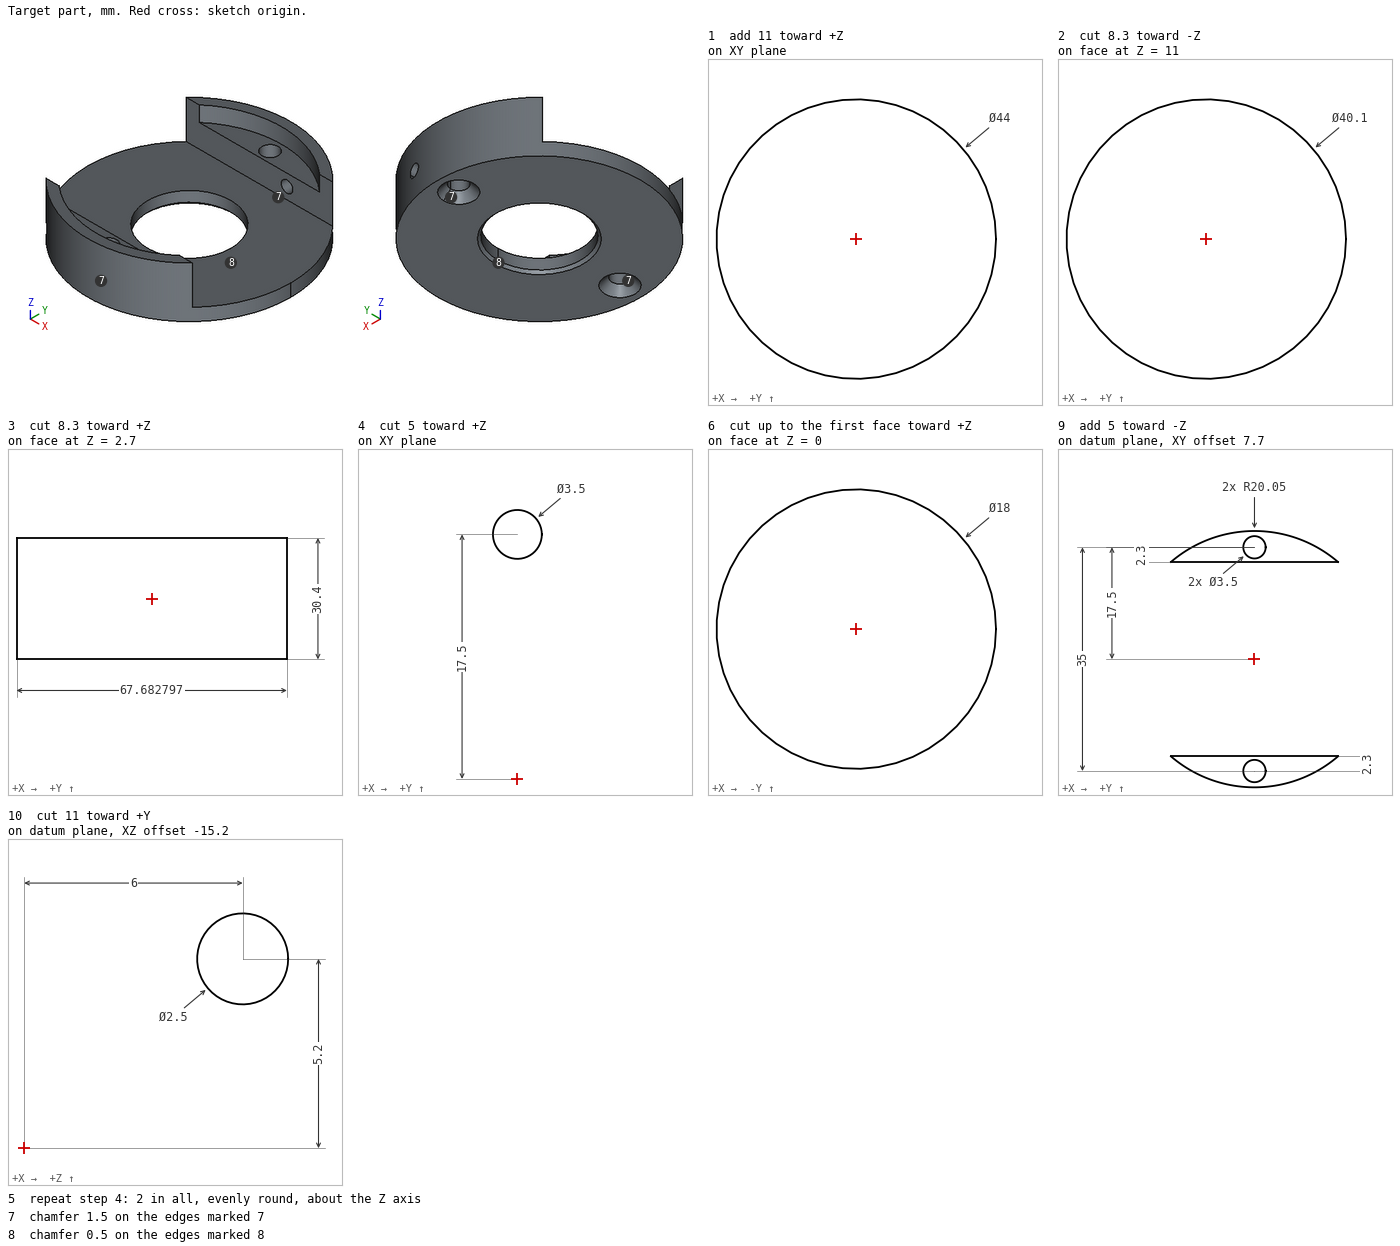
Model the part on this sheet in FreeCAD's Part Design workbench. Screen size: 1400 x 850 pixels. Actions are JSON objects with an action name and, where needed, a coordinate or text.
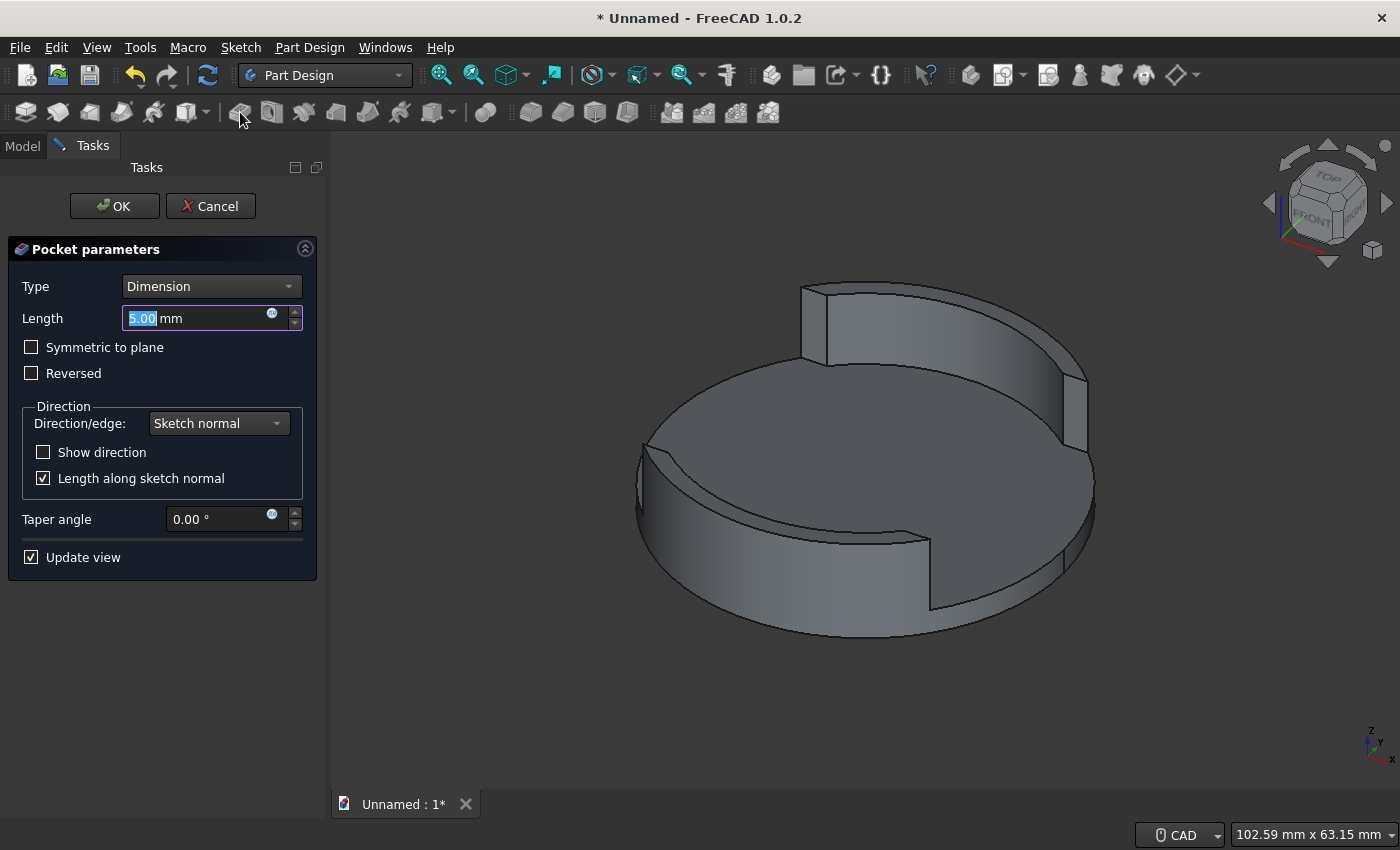
{"action": "type", "text": "5"}
{"action": "key", "text": "Tab"}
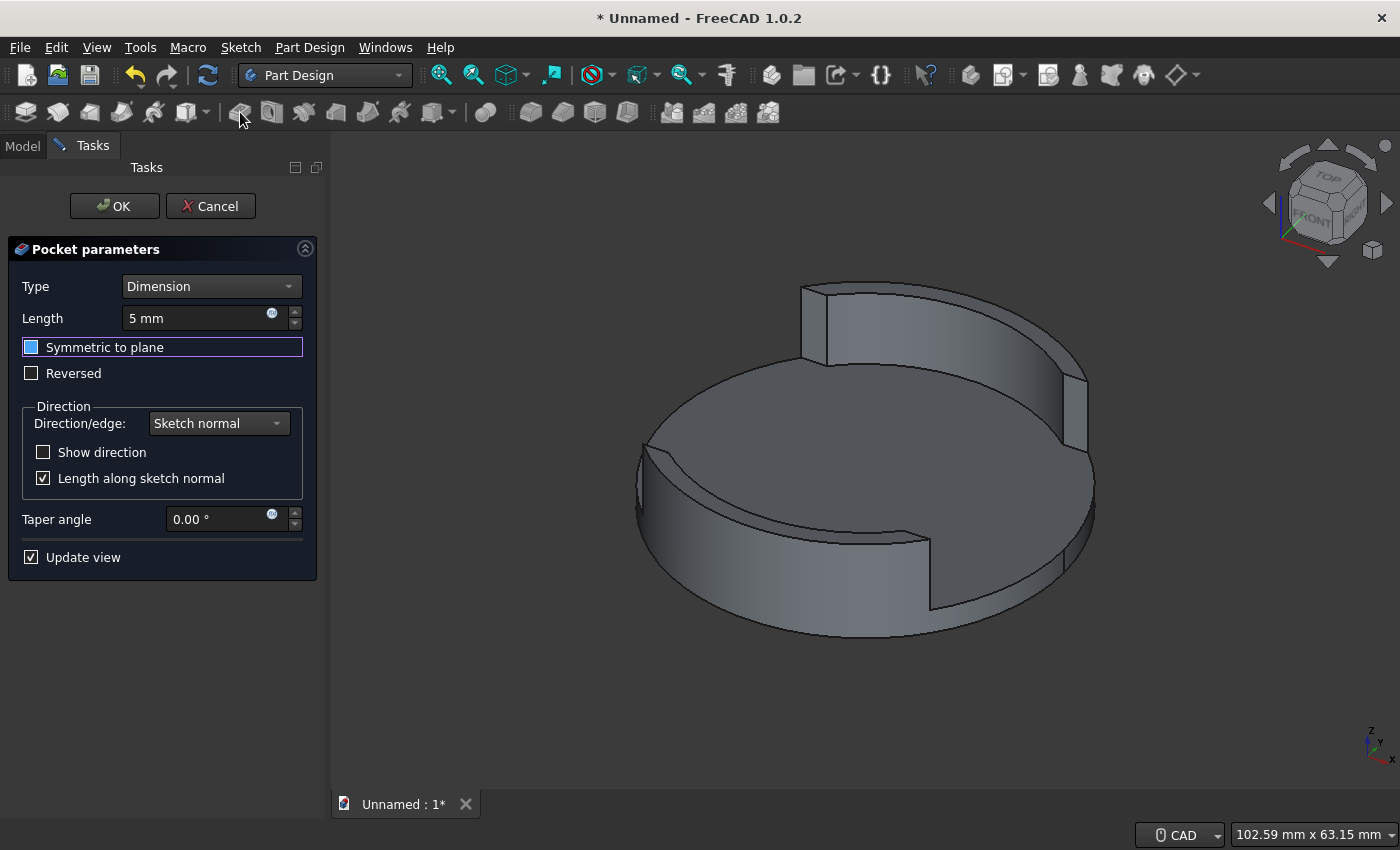
{"action": "left_click", "coordinate": [30, 373]}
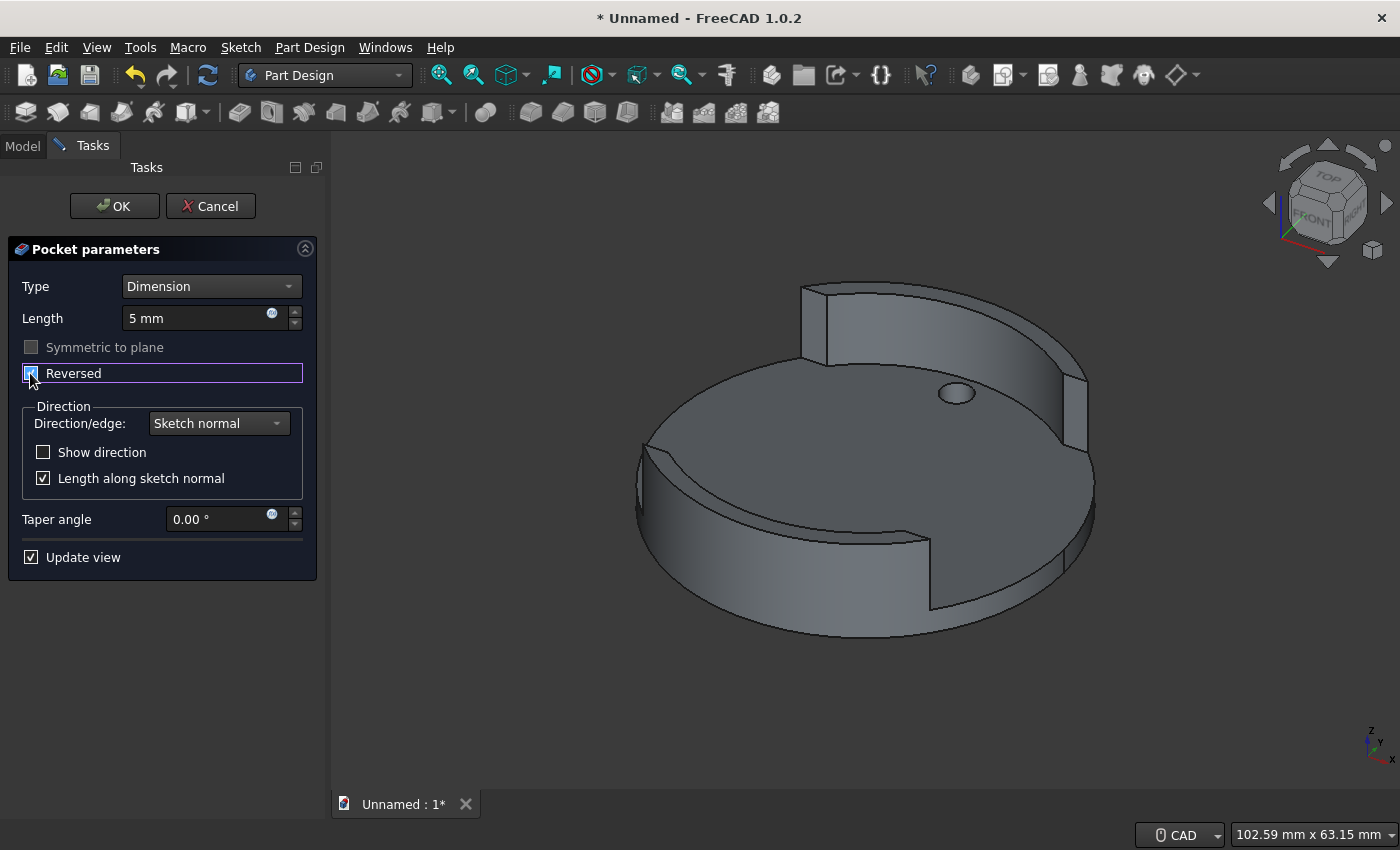
{"action": "left_click", "coordinate": [115, 206]}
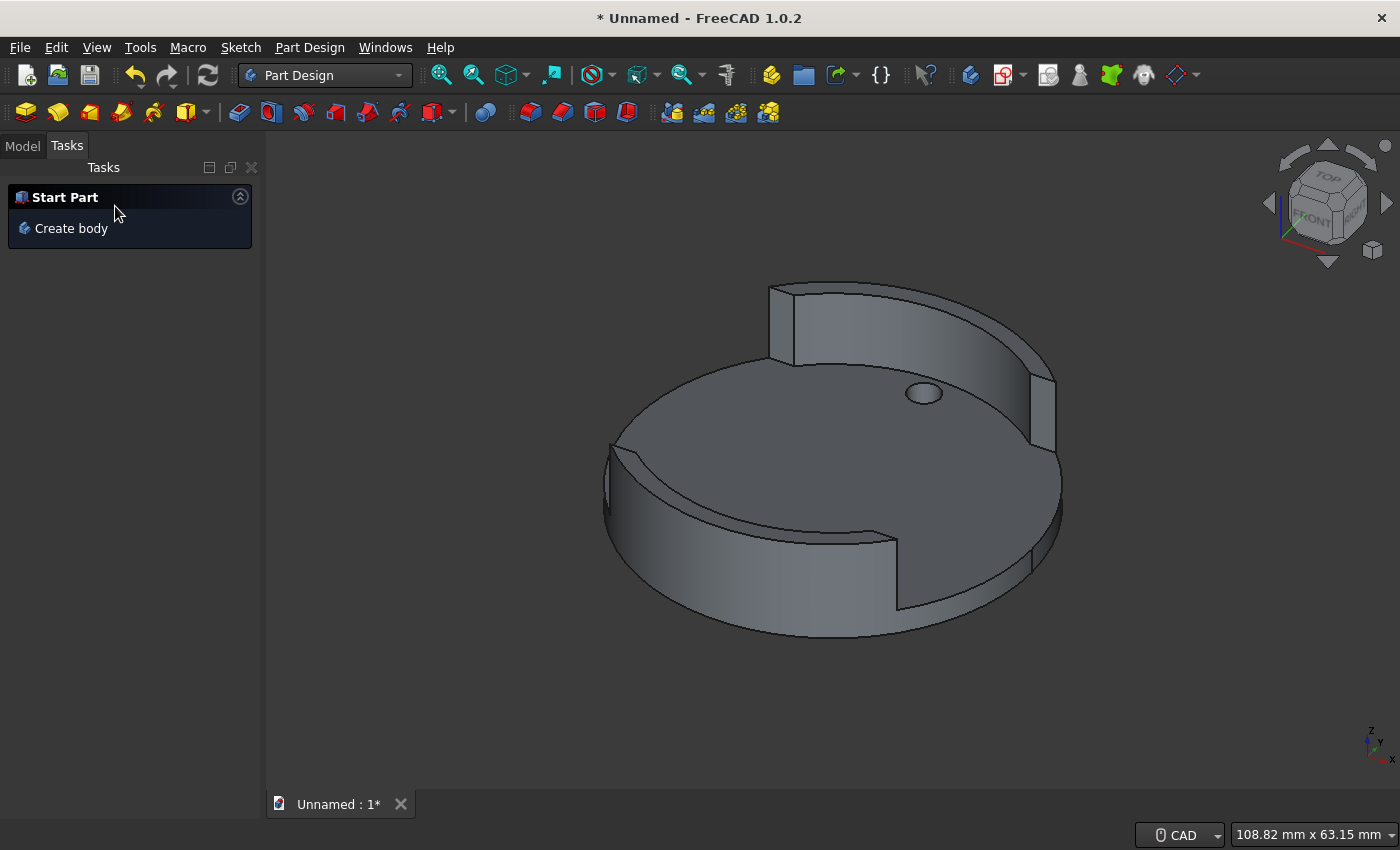
{"action": "left_click", "coordinate": [23, 145]}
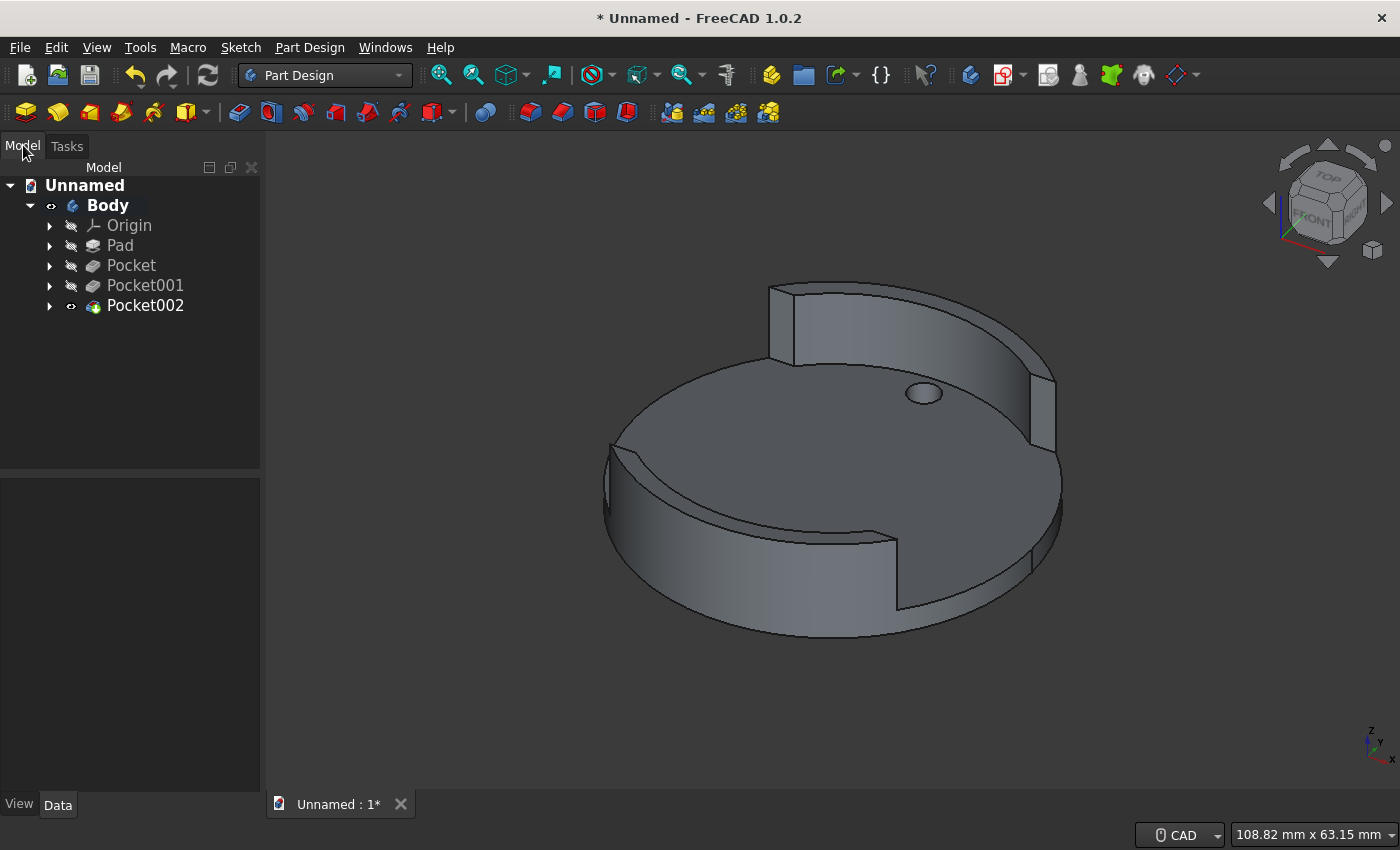
{"action": "left_click", "coordinate": [116, 306]}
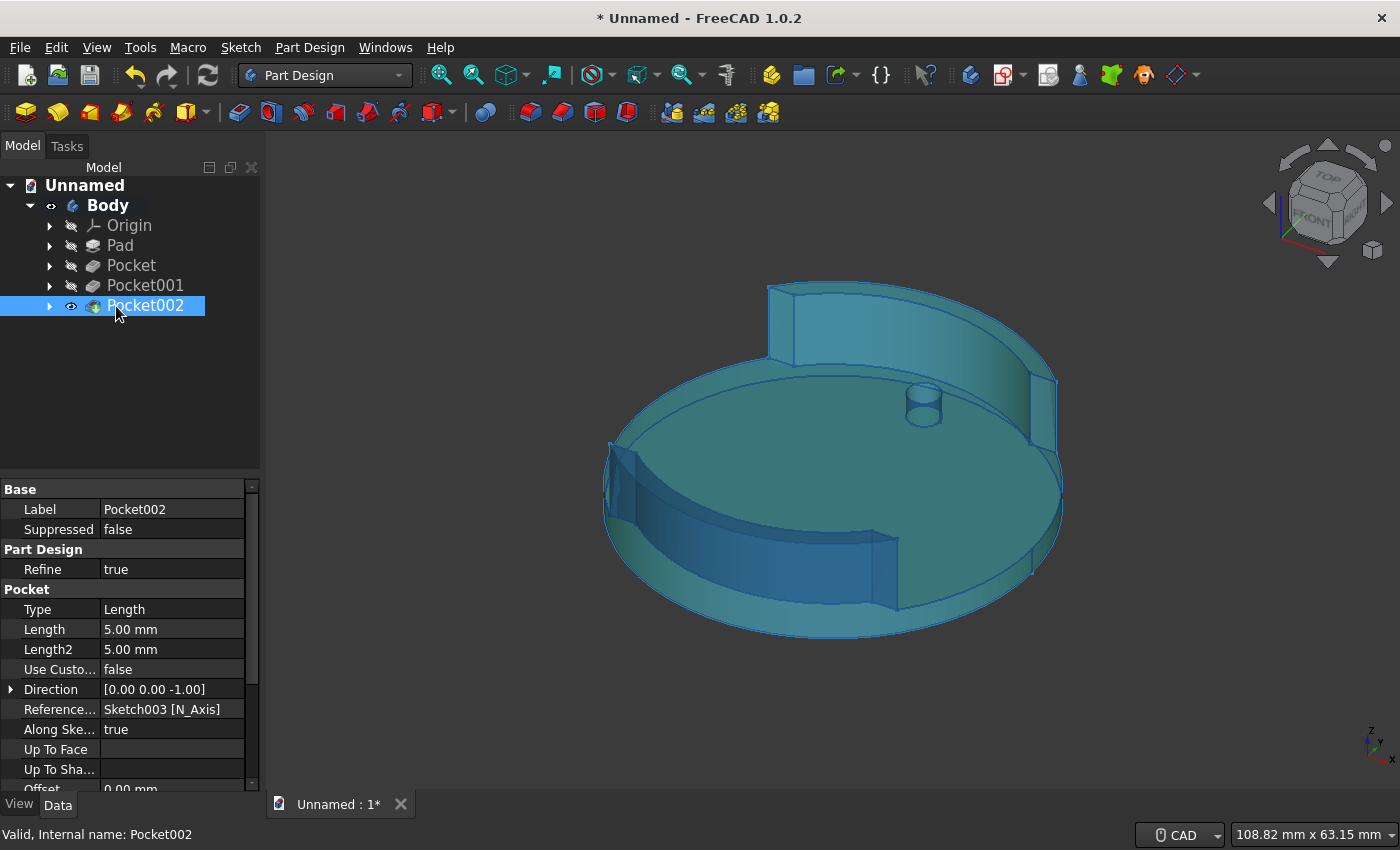
{"action": "left_click", "coordinate": [736, 112]}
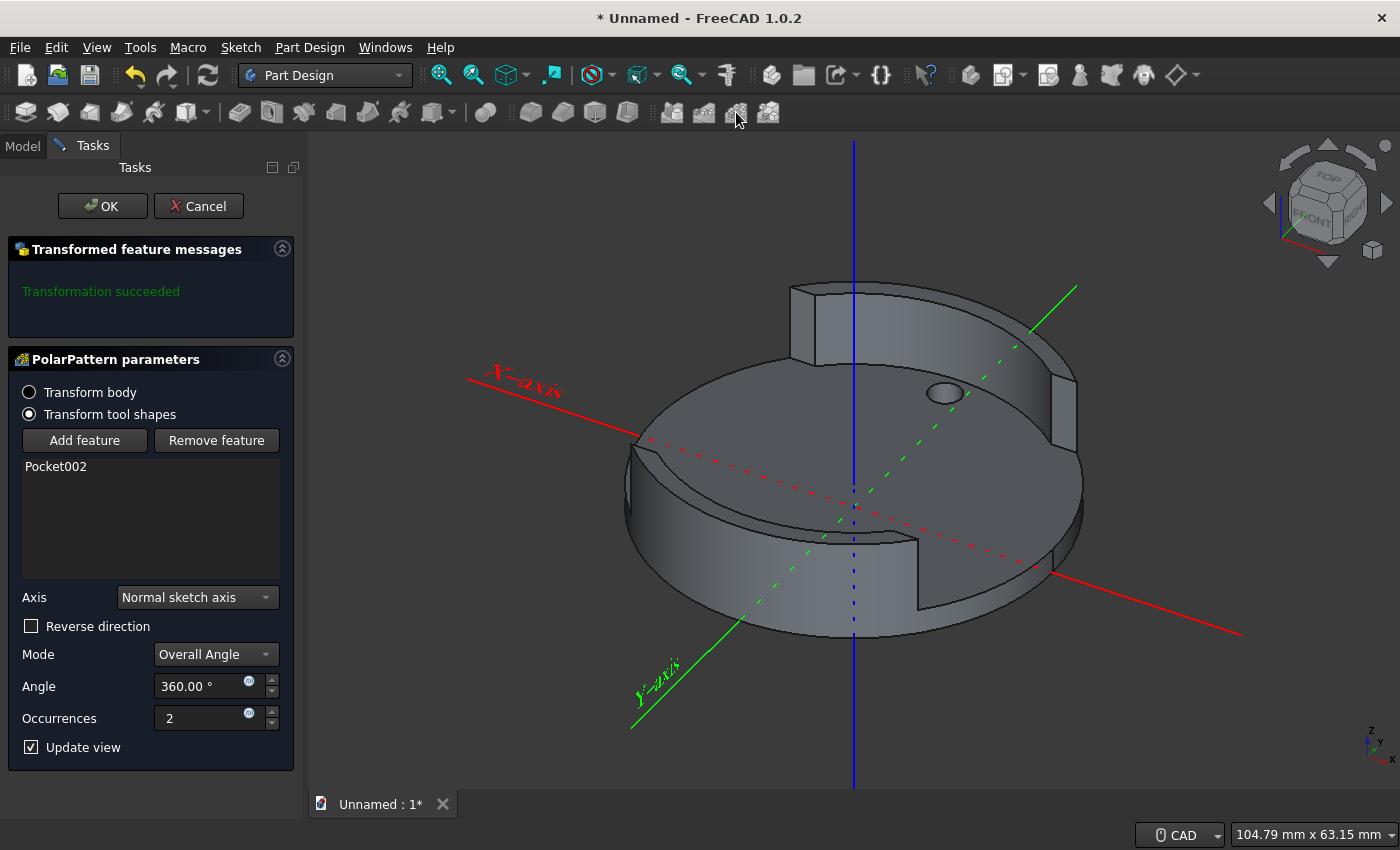
{"action": "left_click", "coordinate": [198, 598]}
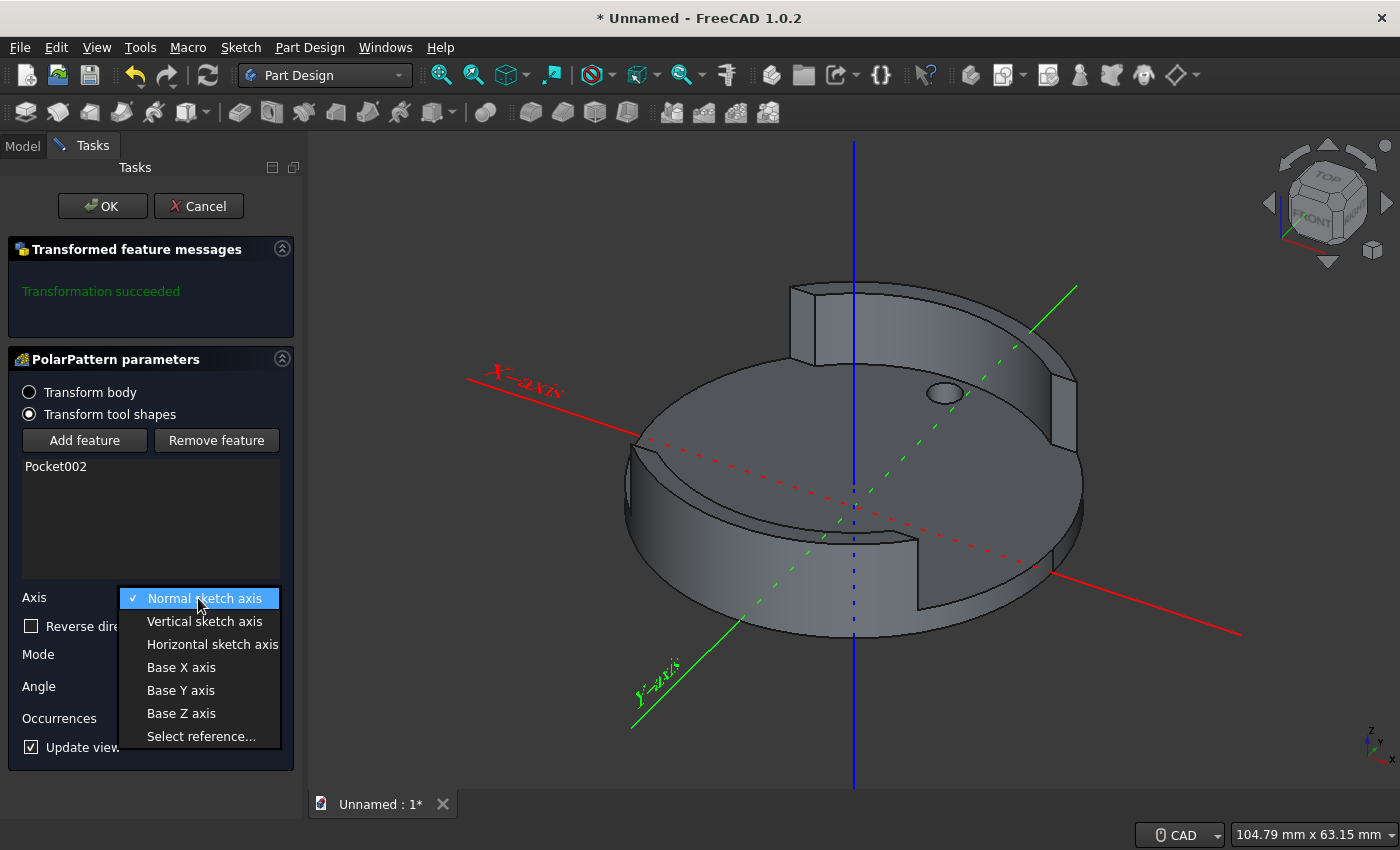
{"action": "left_click", "coordinate": [198, 714]}